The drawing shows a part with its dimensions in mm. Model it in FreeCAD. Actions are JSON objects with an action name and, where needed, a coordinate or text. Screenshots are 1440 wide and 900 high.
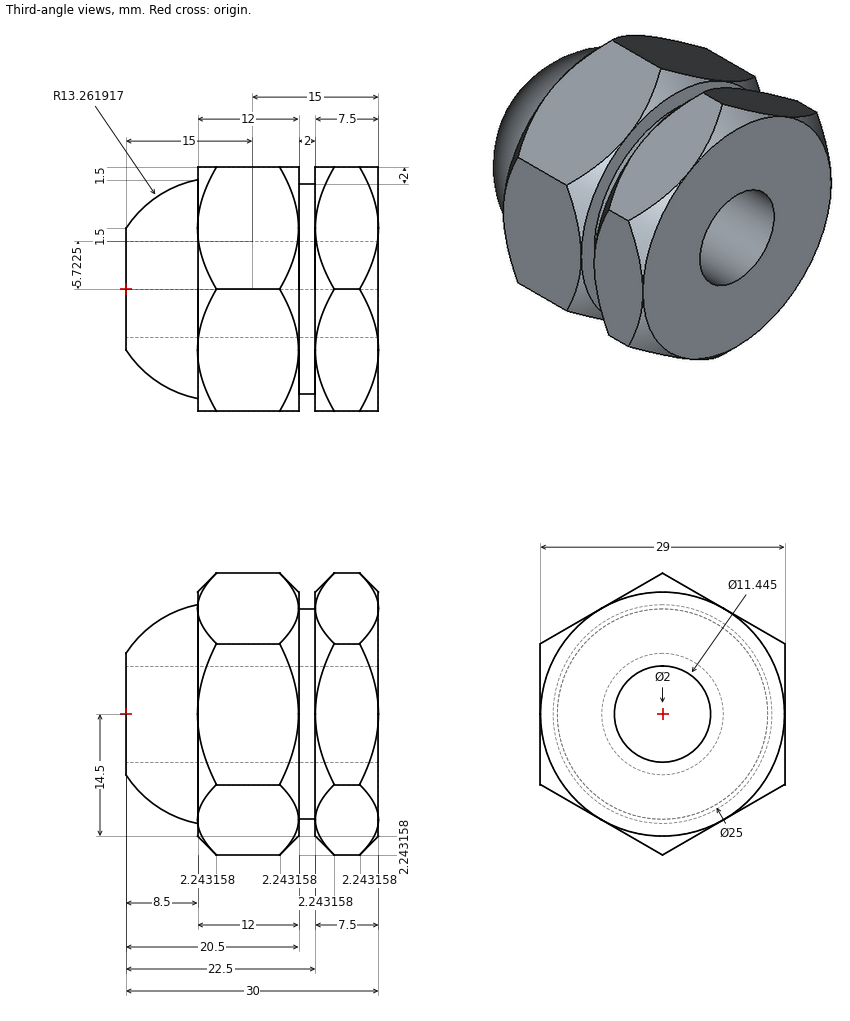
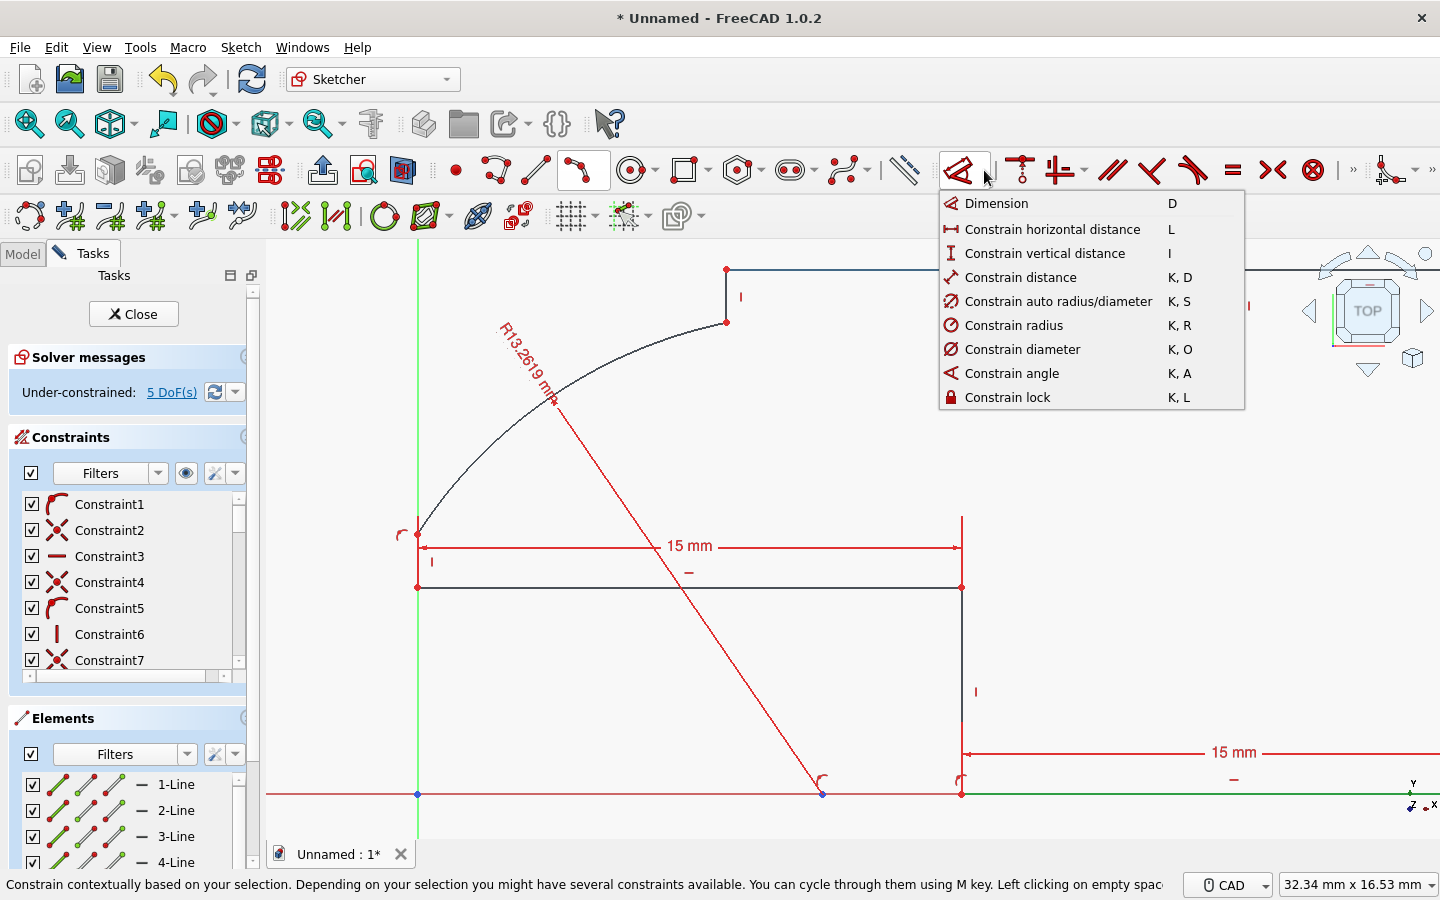
{"action": "left_click", "coordinate": [1092, 229]}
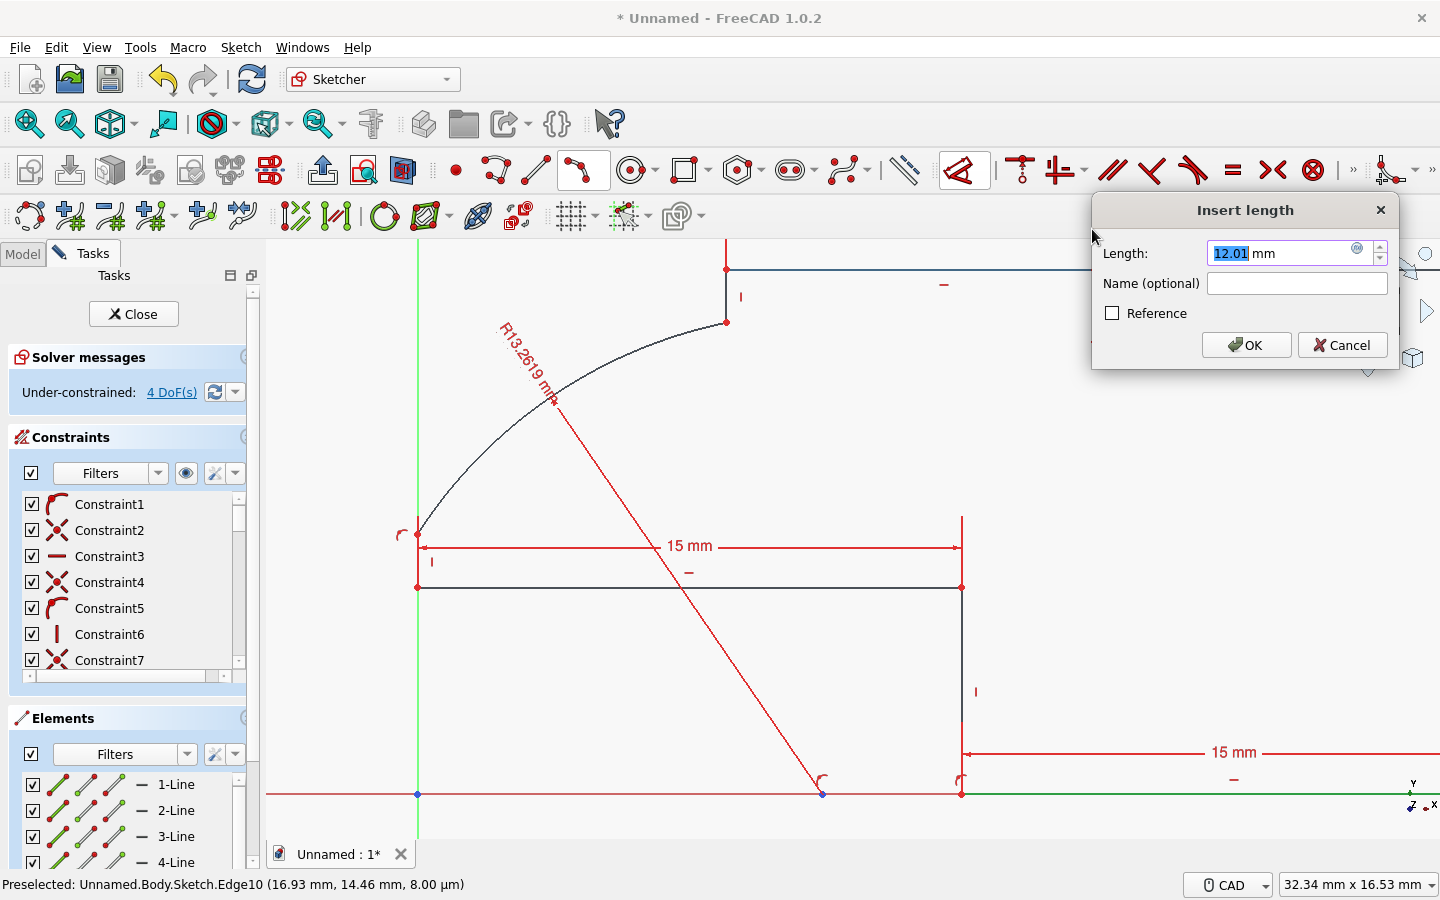
{"action": "type", "text": "12"}
{"action": "key", "text": "Return"}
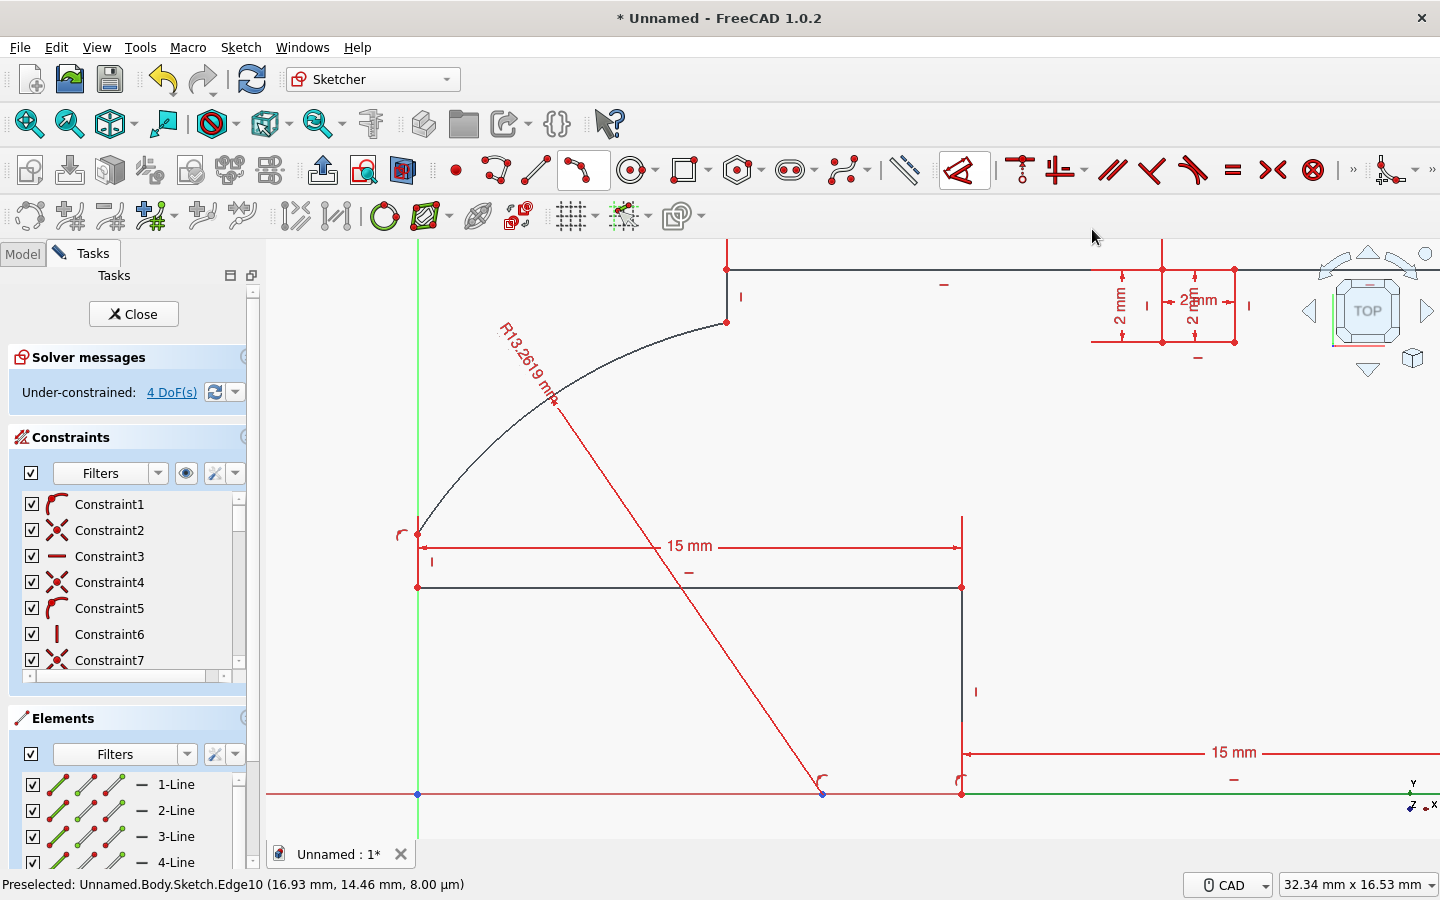
{"action": "left_click", "coordinate": [418, 550]}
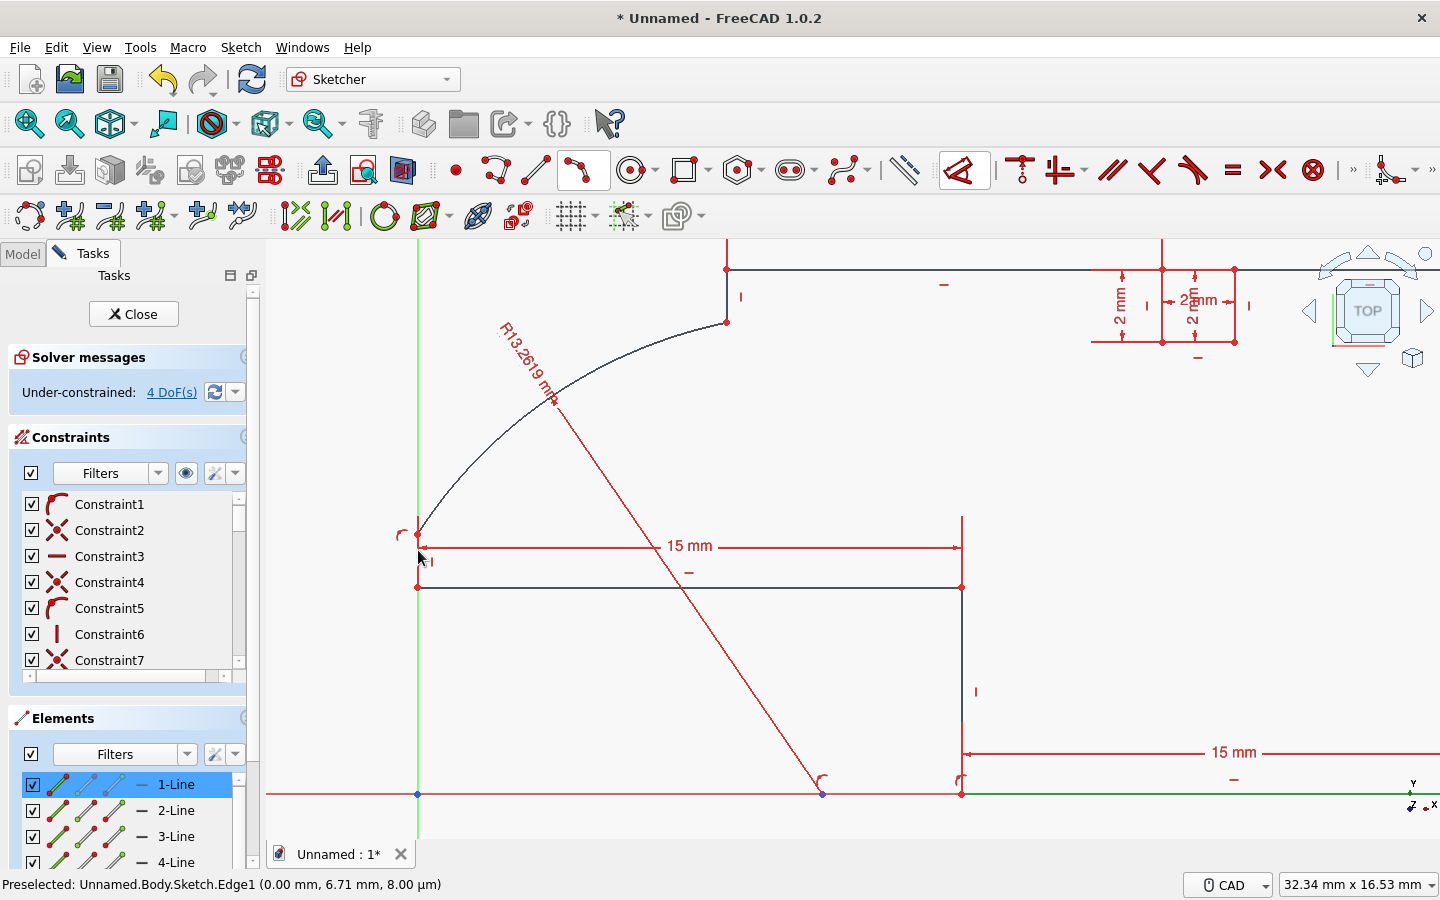
{"action": "key", "text": "i"}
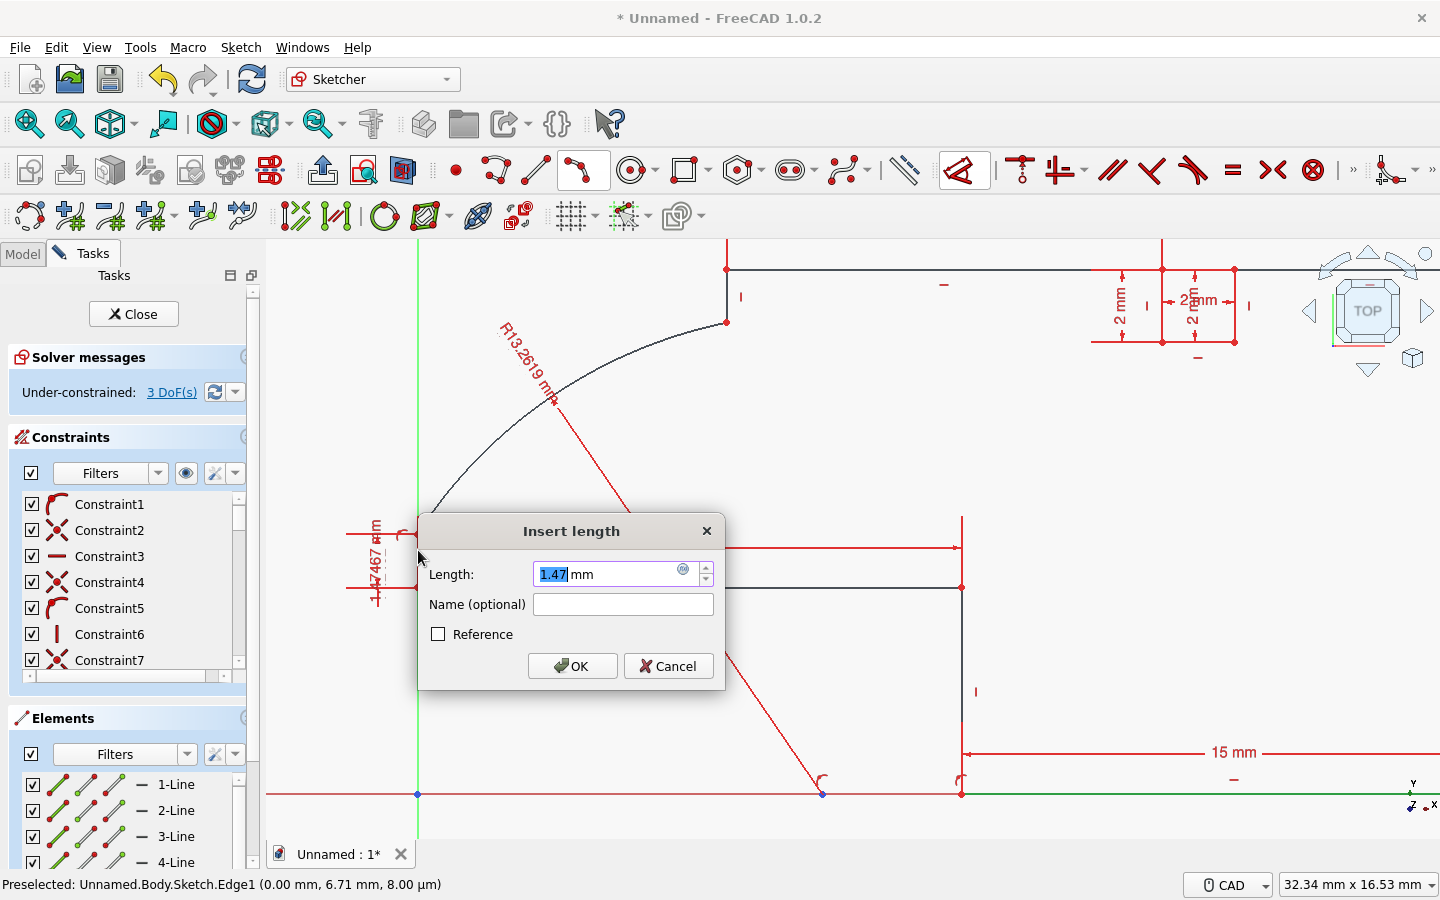
{"action": "type", "text": "1.5"}
{"action": "key", "text": "Return"}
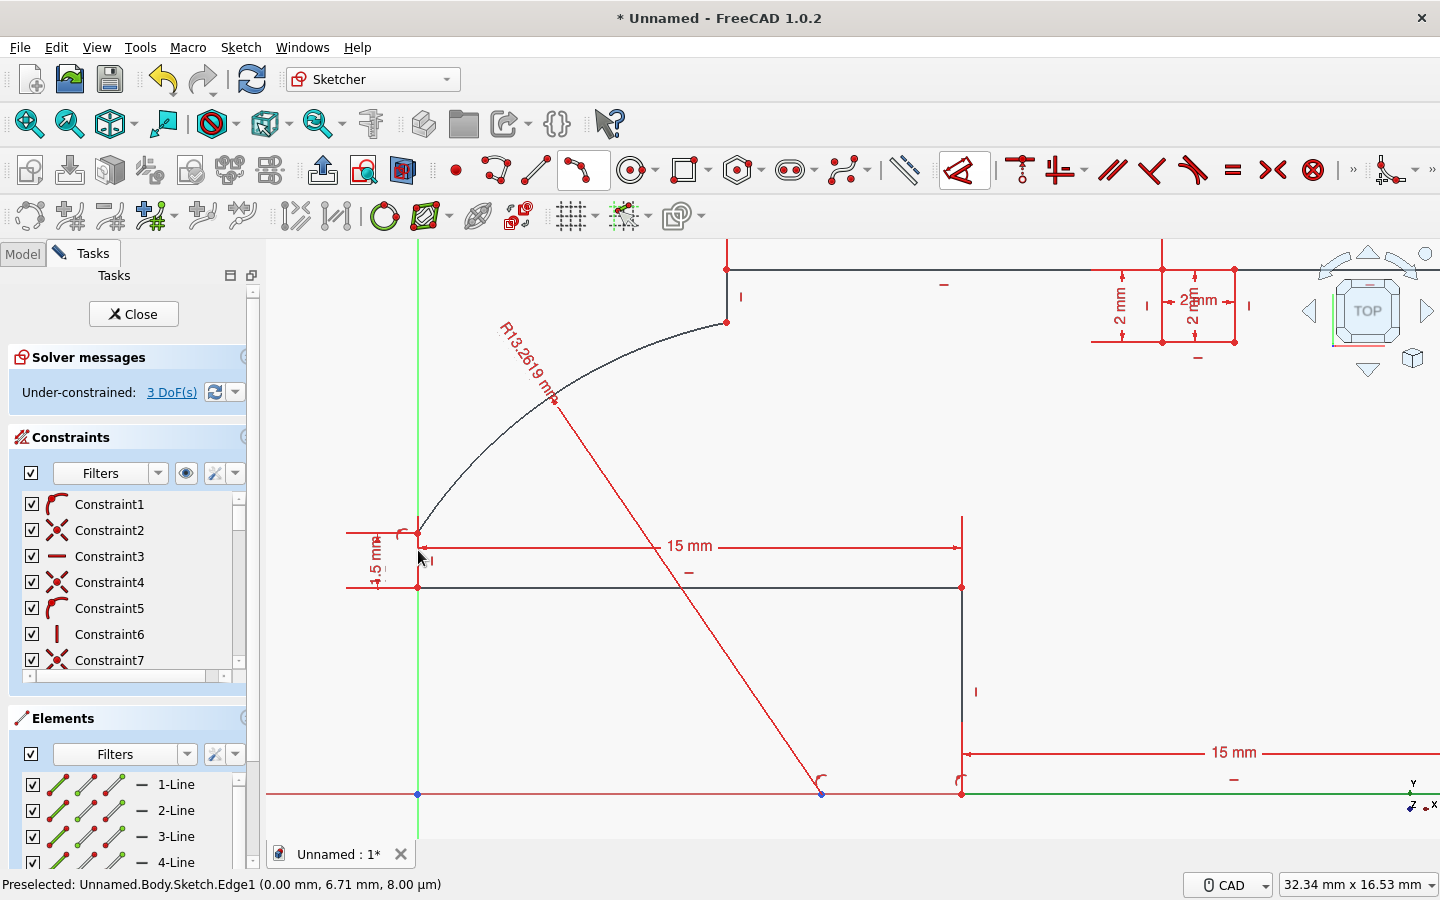
{"action": "scroll", "coordinate": [424, 555], "scroll_direction": "down", "scroll_amount": 2}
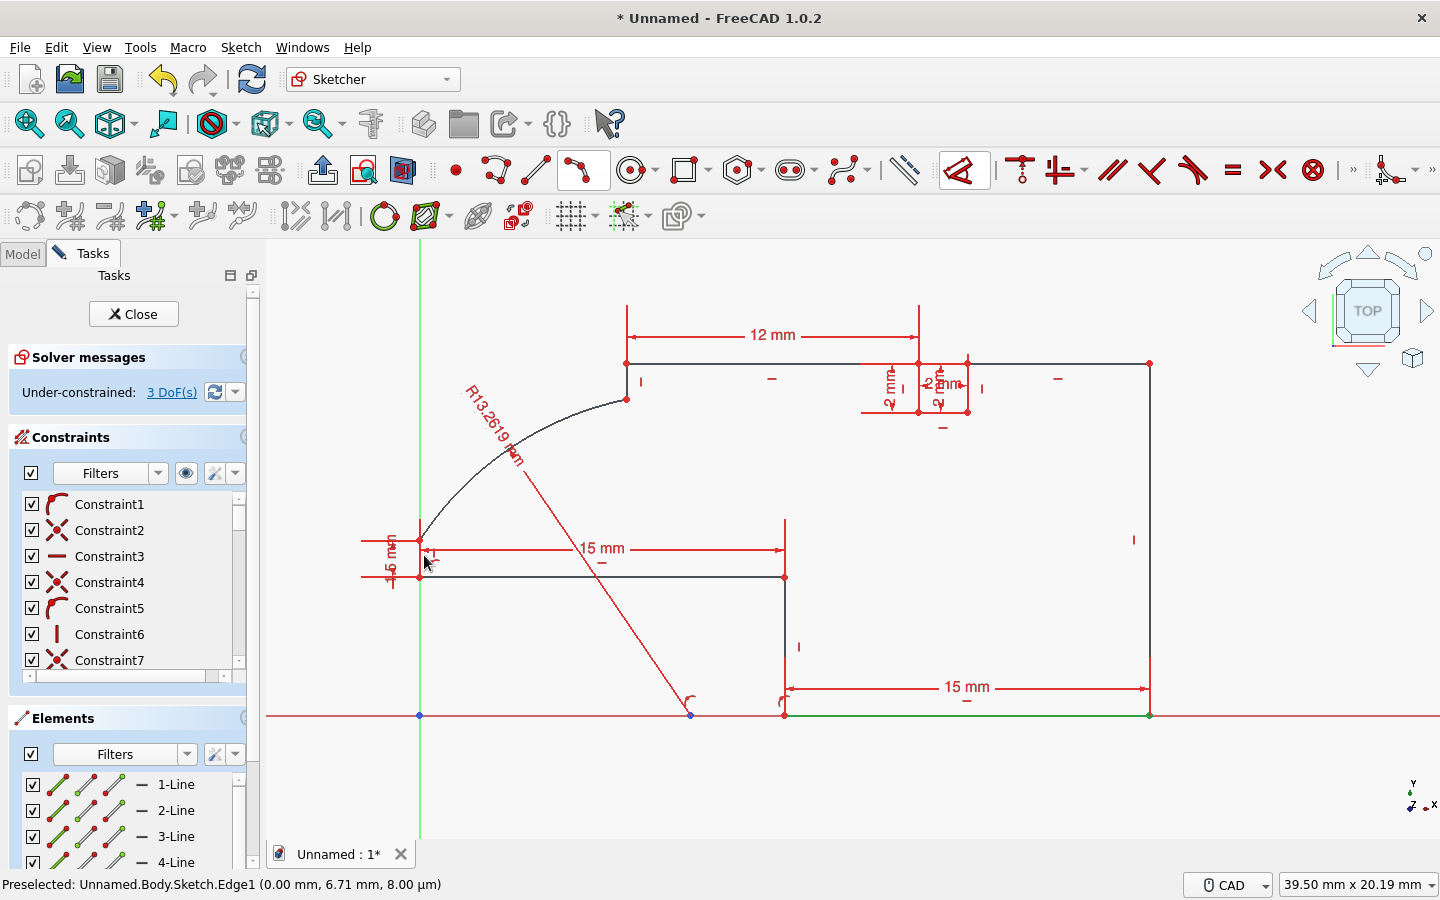
{"action": "left_click", "coordinate": [1095, 364]}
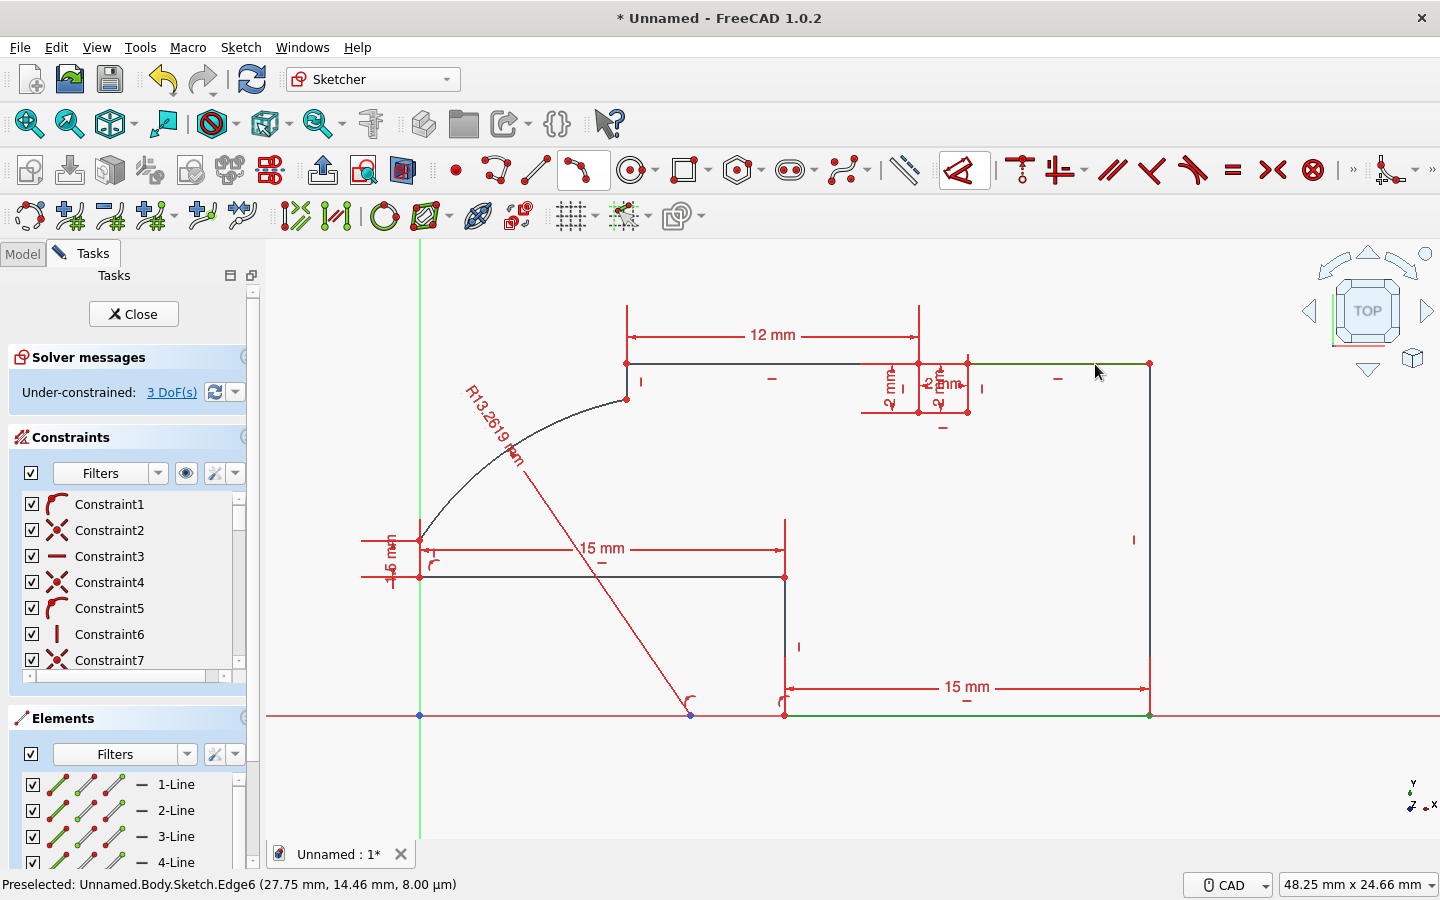
{"action": "left_click", "coordinate": [984, 170]}